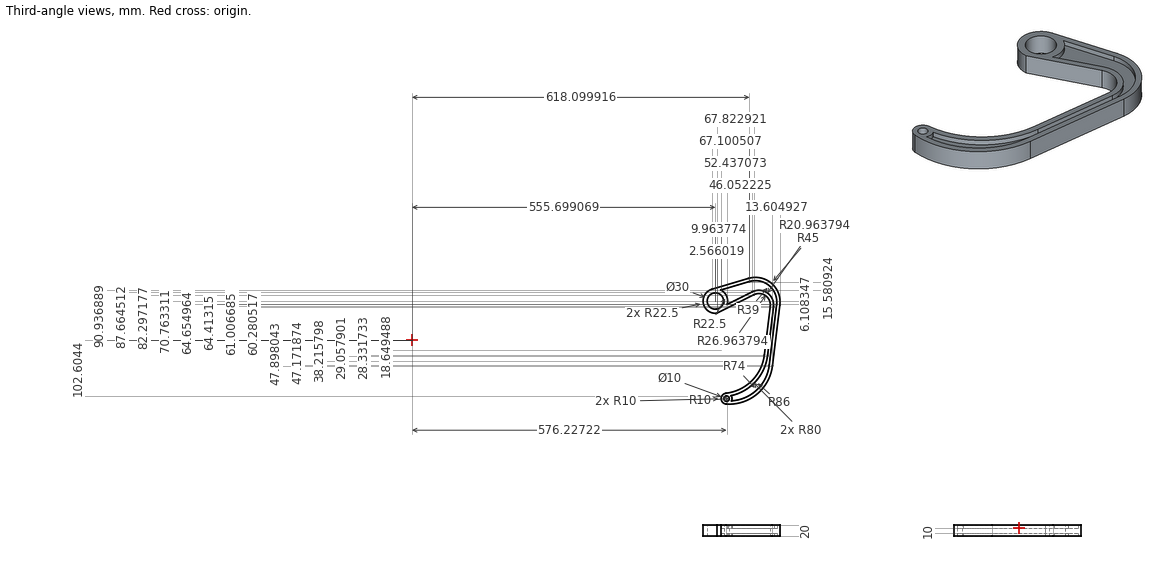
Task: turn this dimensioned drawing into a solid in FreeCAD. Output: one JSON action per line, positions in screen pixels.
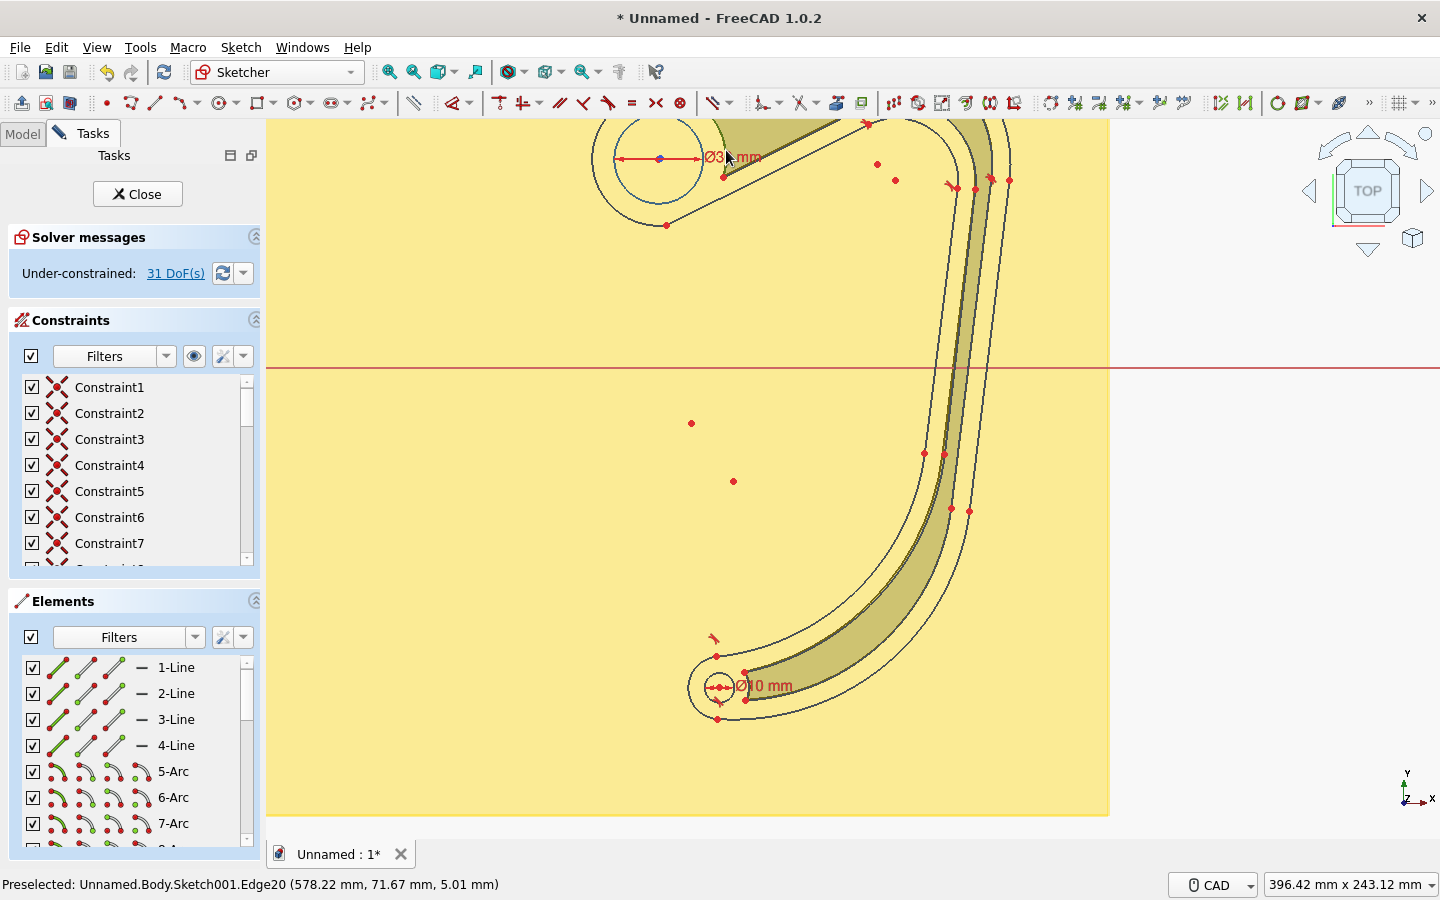
{"action": "left_click", "coordinate": [500, 104]}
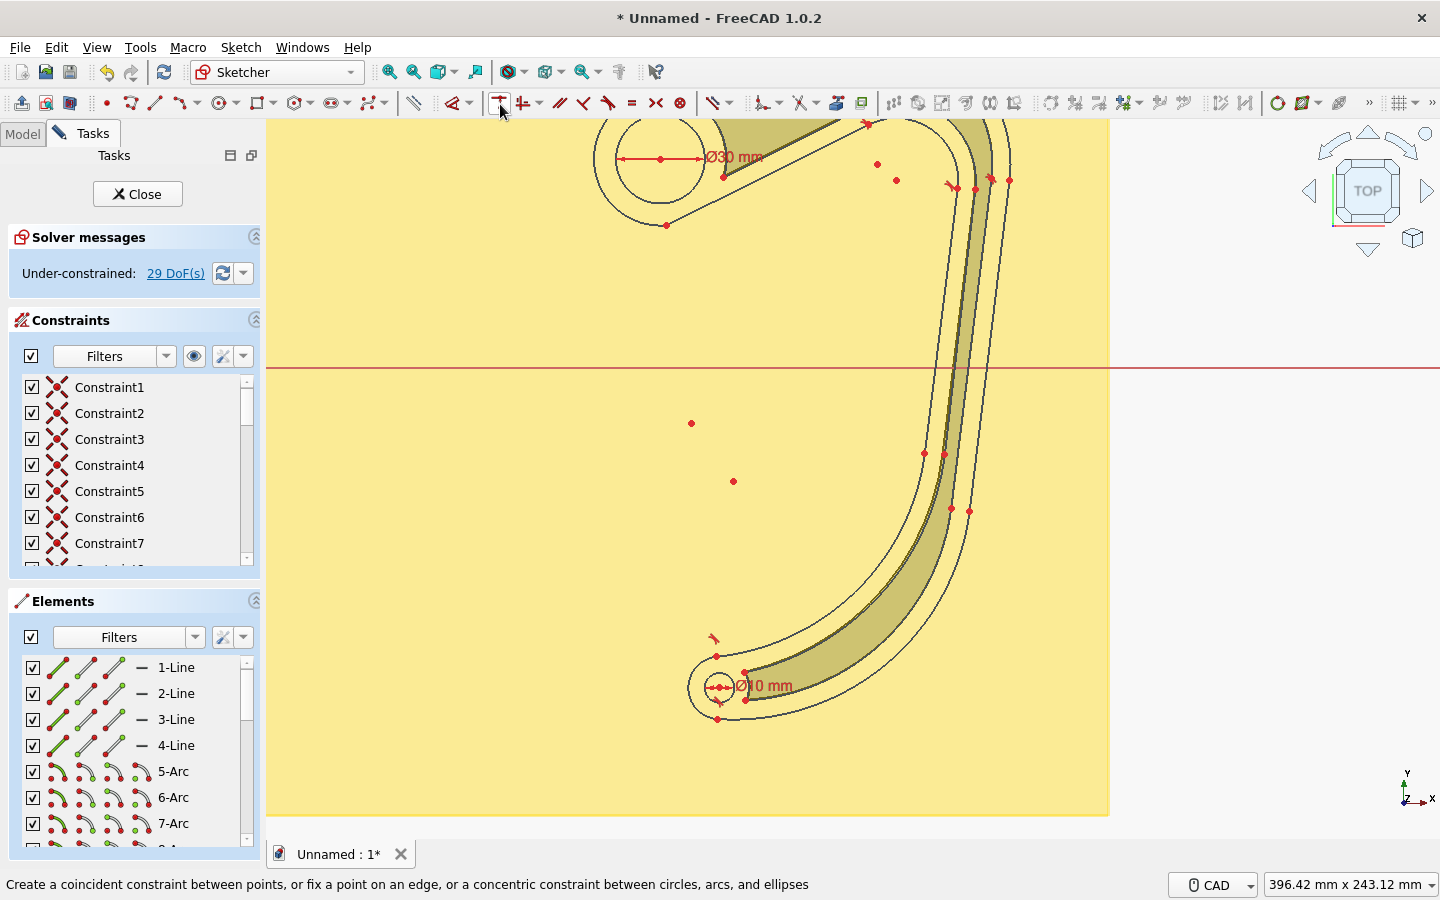
{"action": "left_click", "coordinate": [806, 629]}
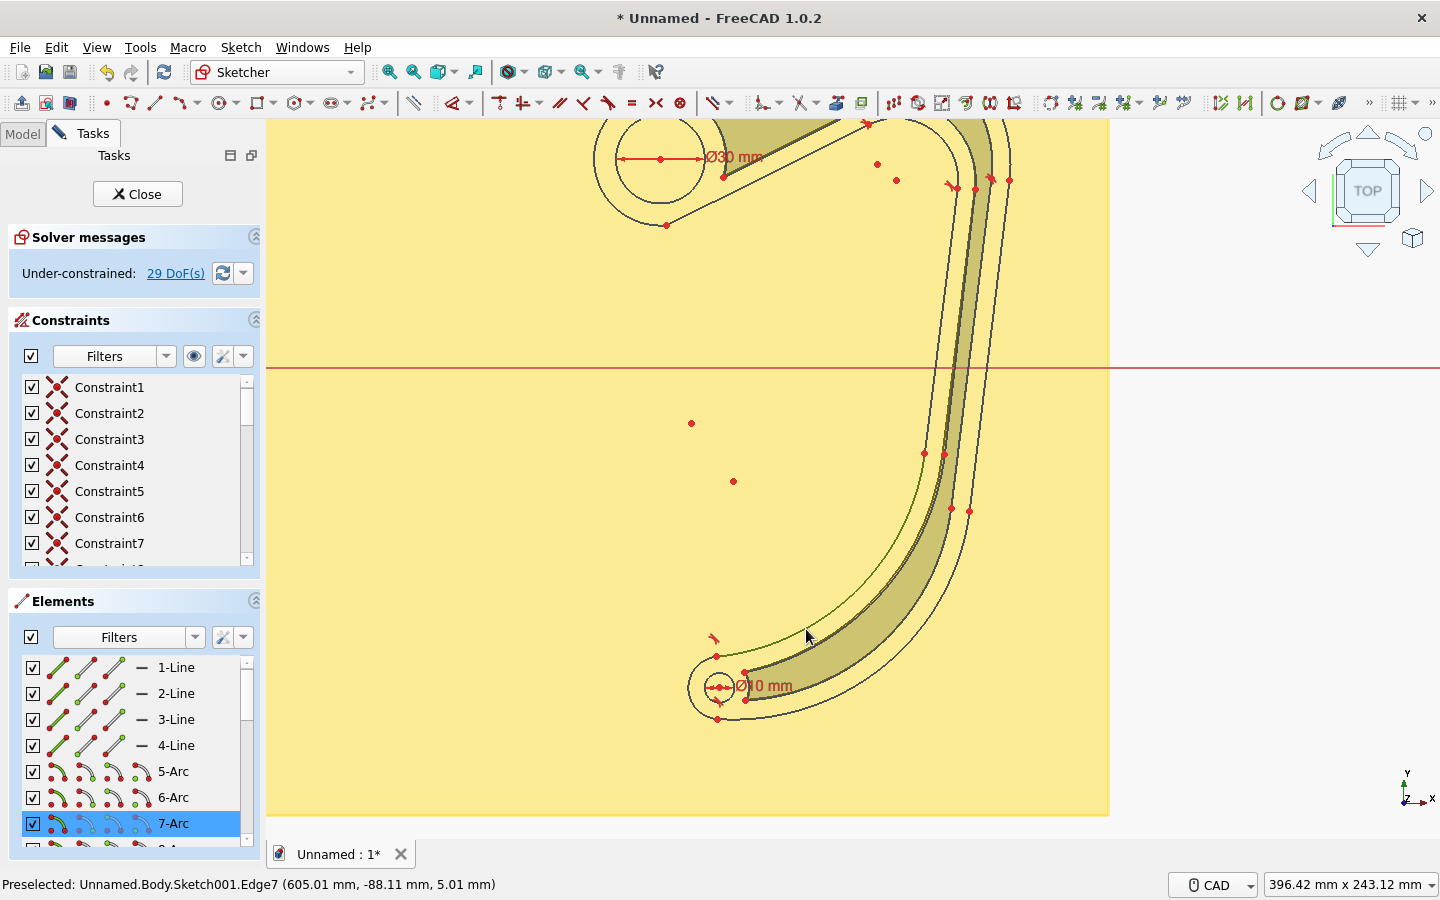
{"action": "left_click", "coordinate": [823, 702]}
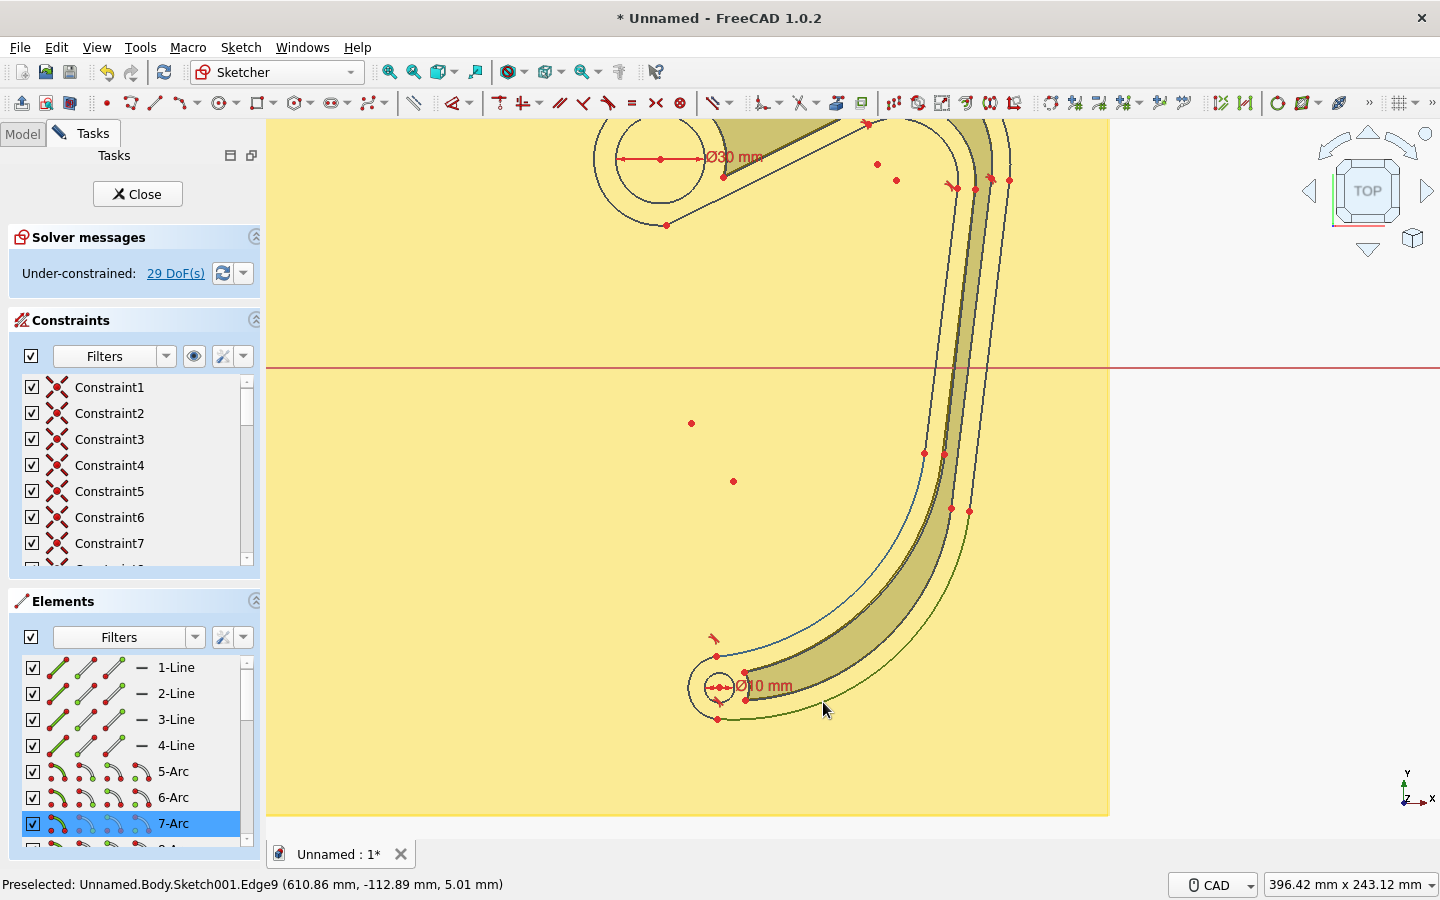
{"action": "left_click", "coordinate": [632, 104]}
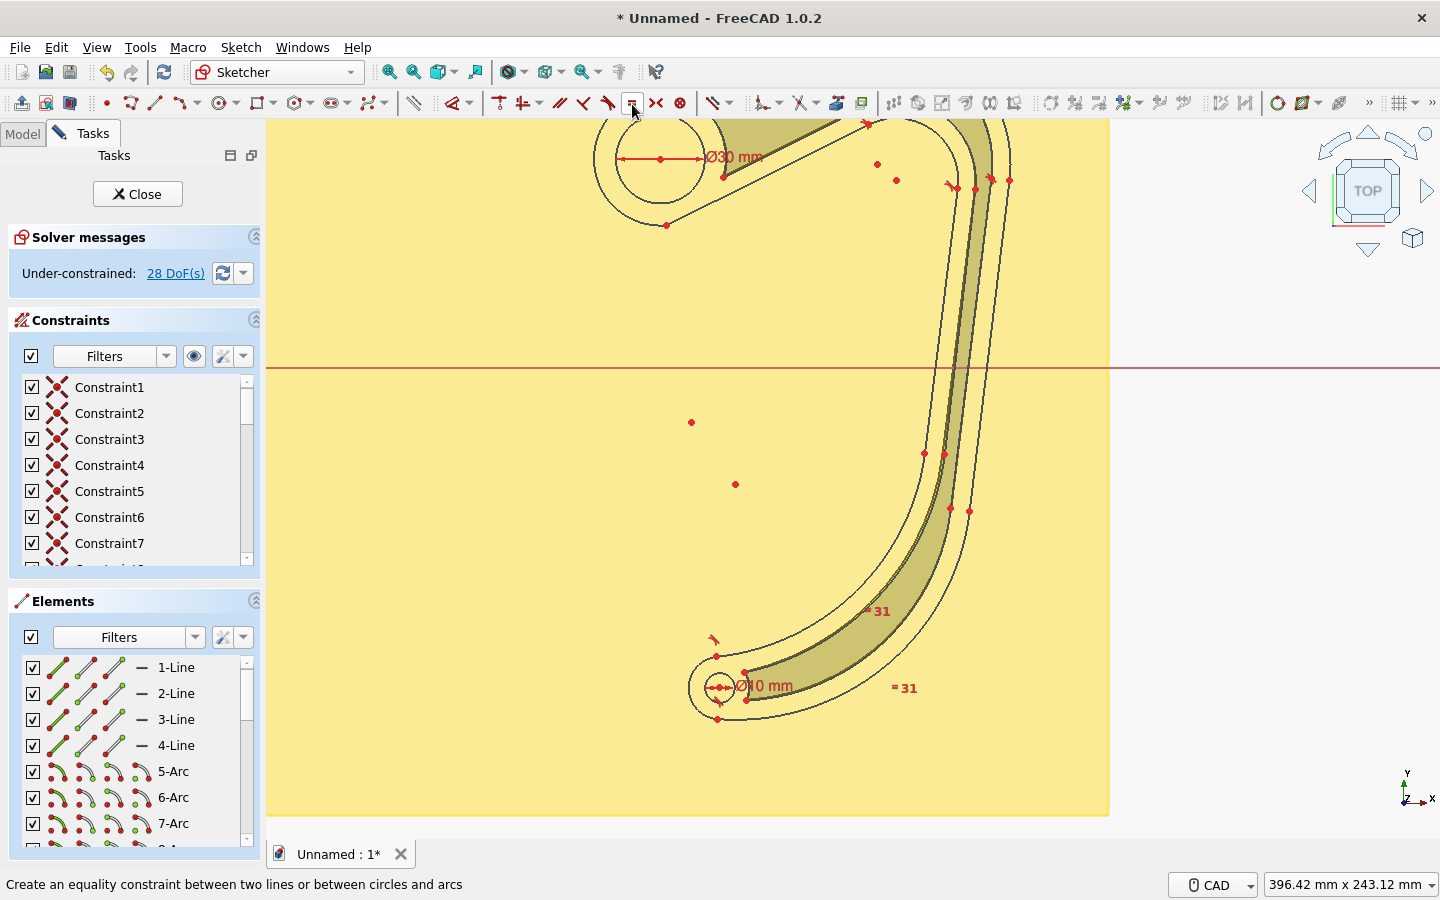
{"action": "left_click", "coordinate": [694, 671]}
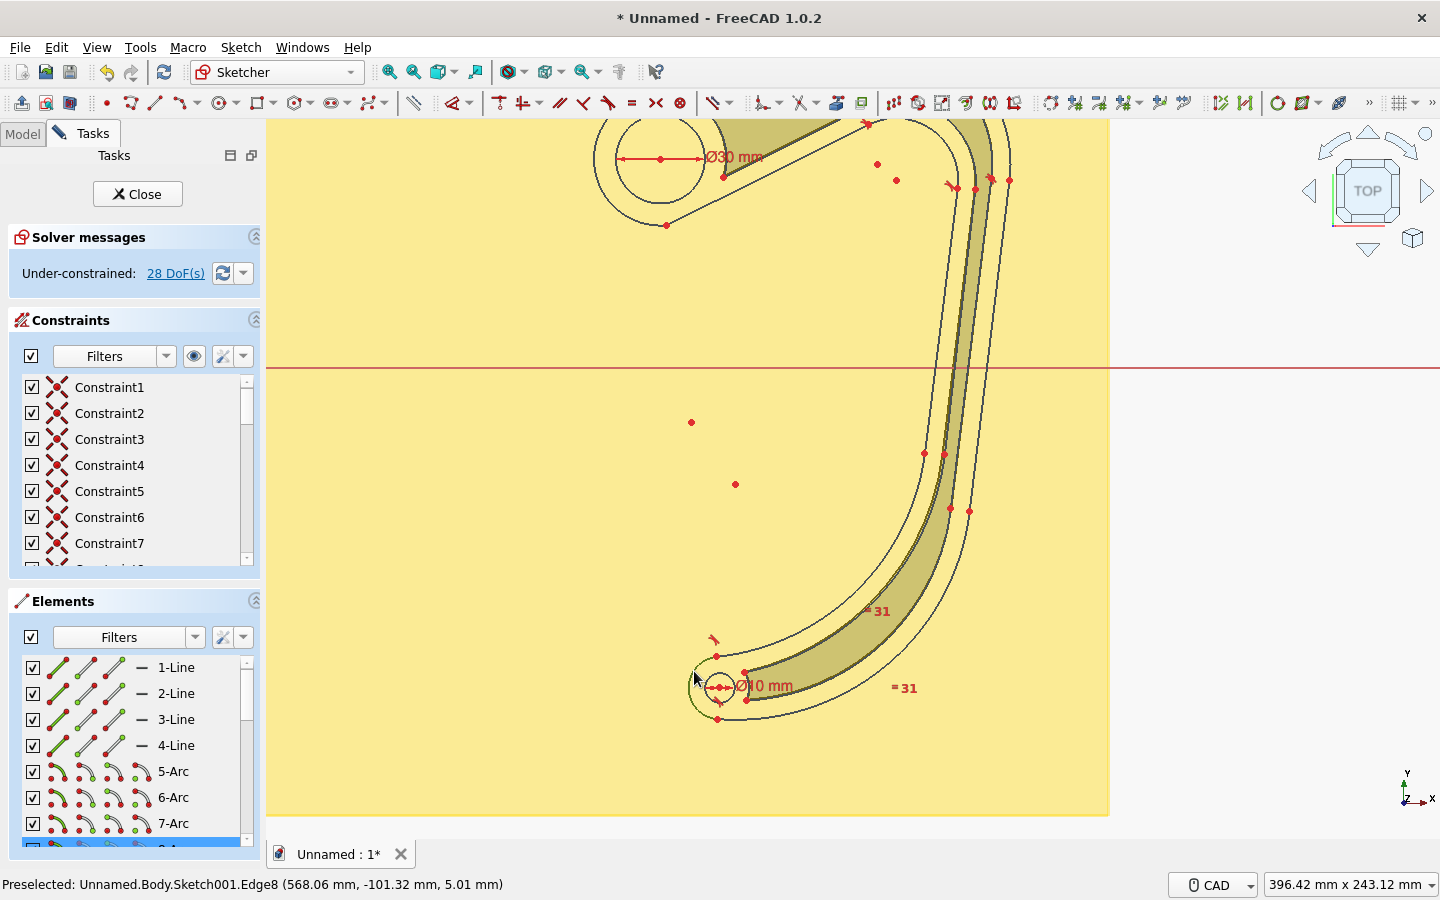
{"action": "left_click", "coordinate": [748, 681]}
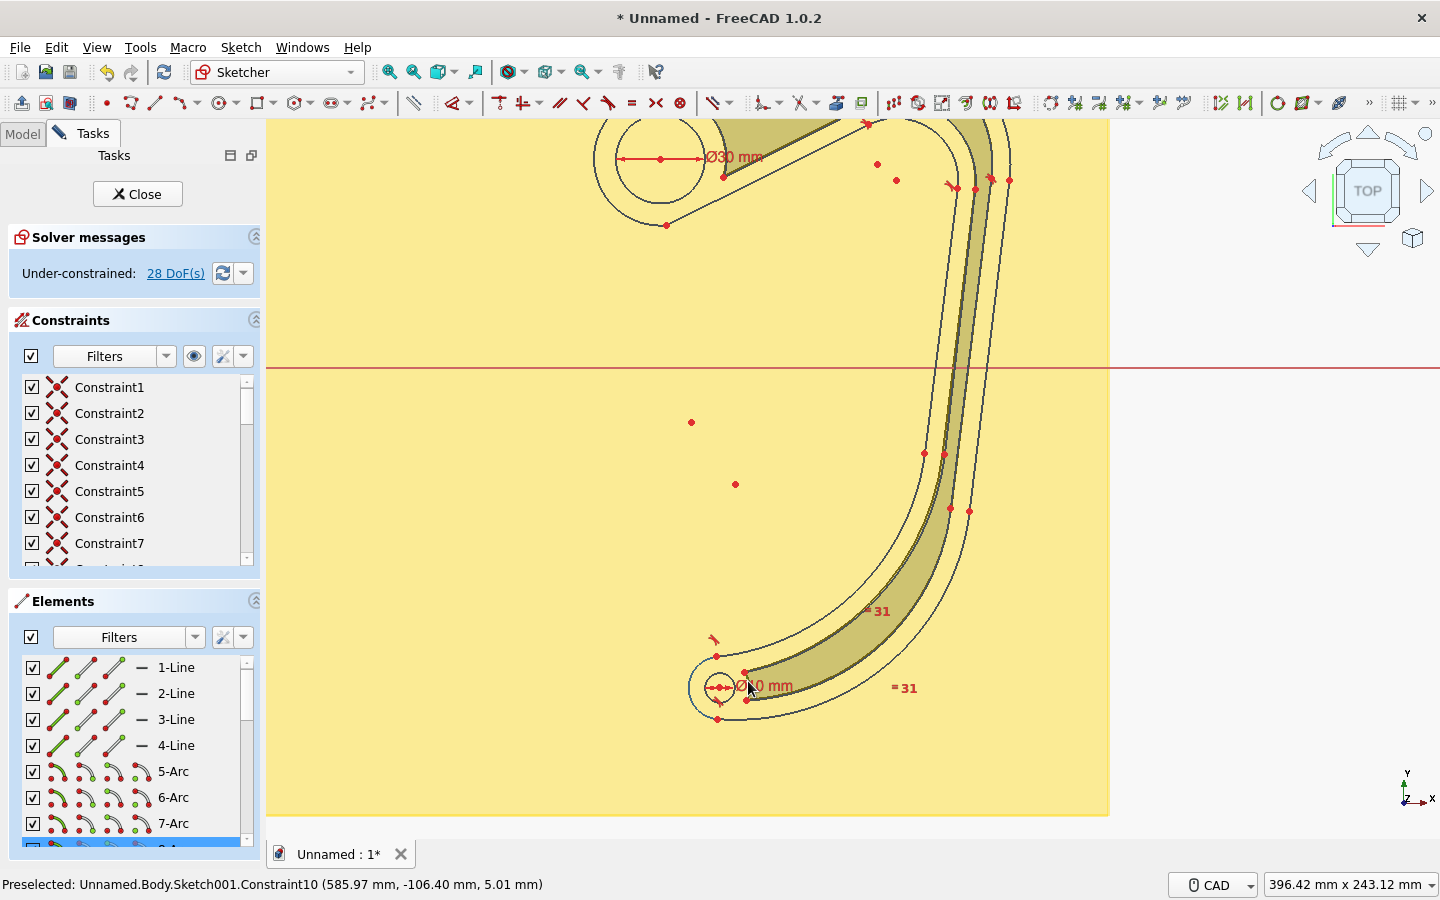
{"action": "key", "text": "e"}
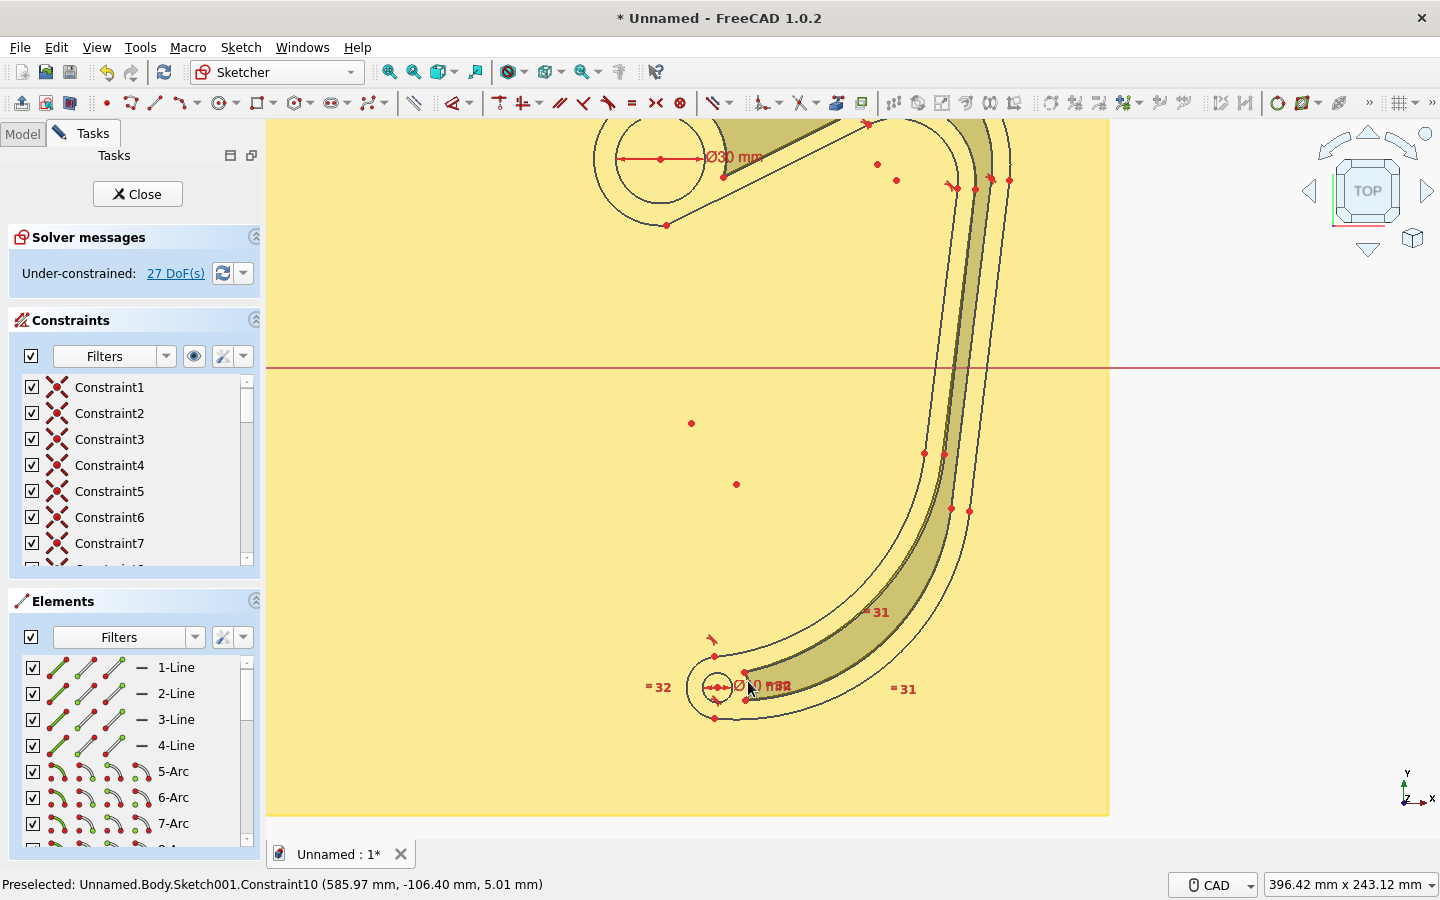
{"action": "left_click", "coordinate": [613, 206]}